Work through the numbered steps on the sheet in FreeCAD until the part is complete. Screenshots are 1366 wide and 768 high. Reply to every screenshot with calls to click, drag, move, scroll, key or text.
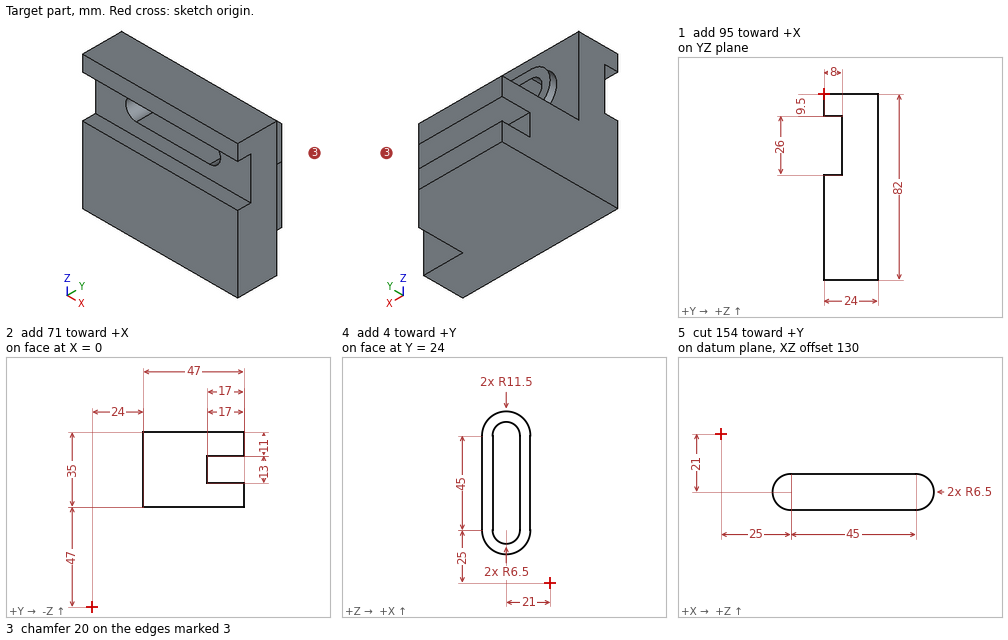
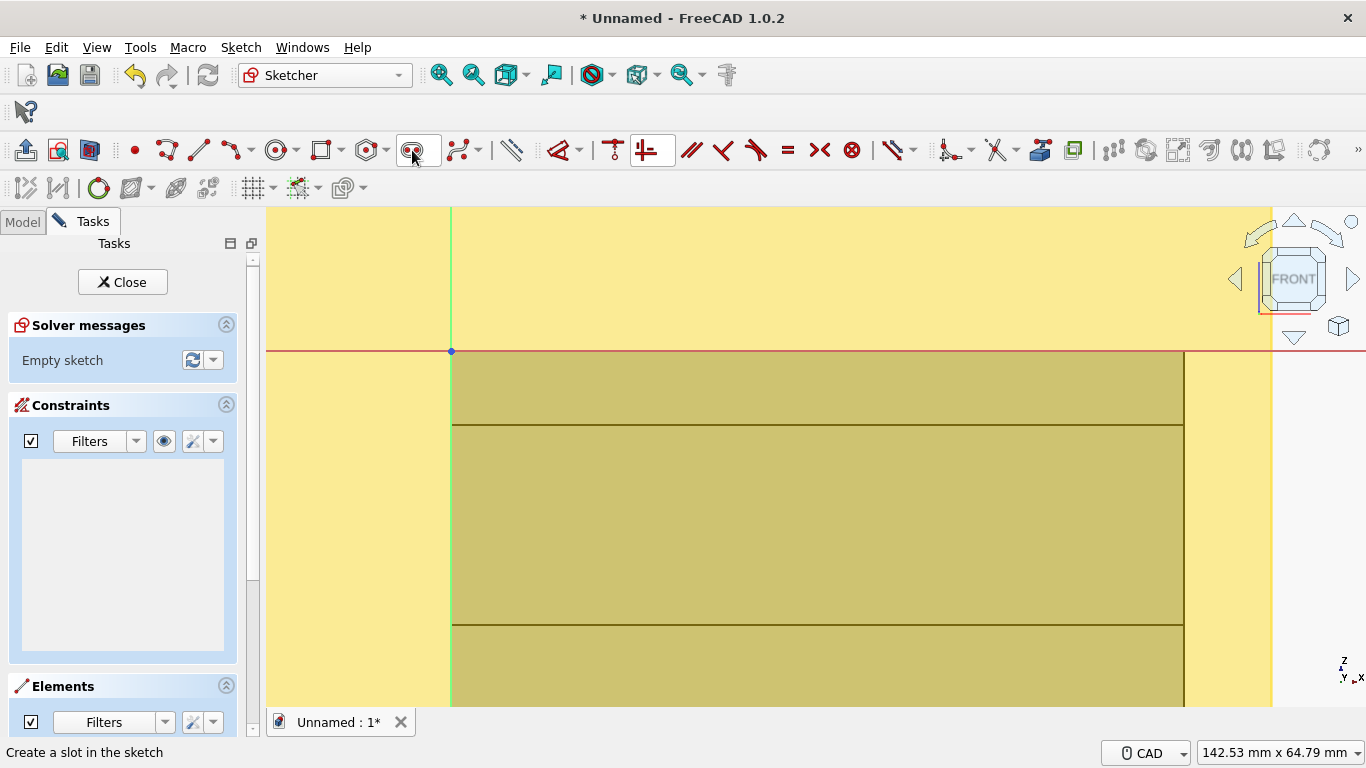
click(644, 513)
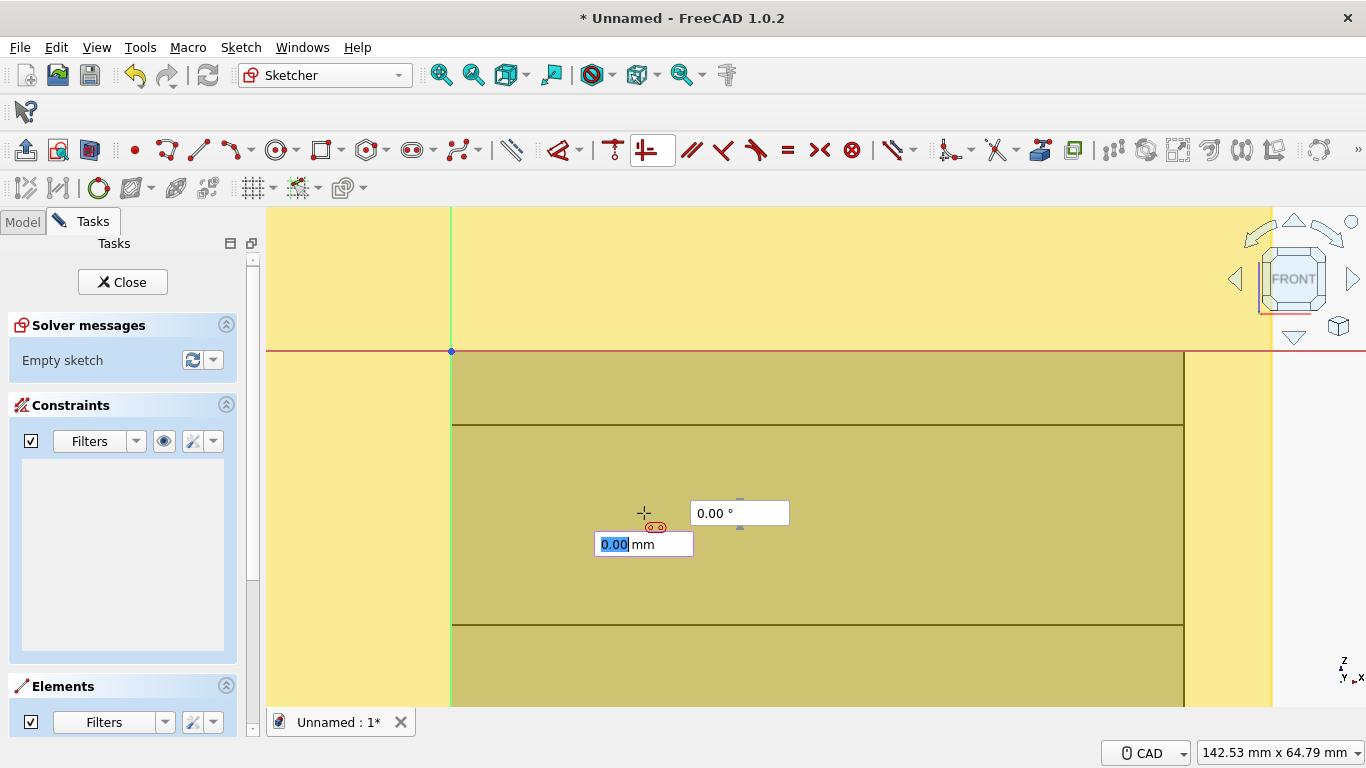
click(991, 513)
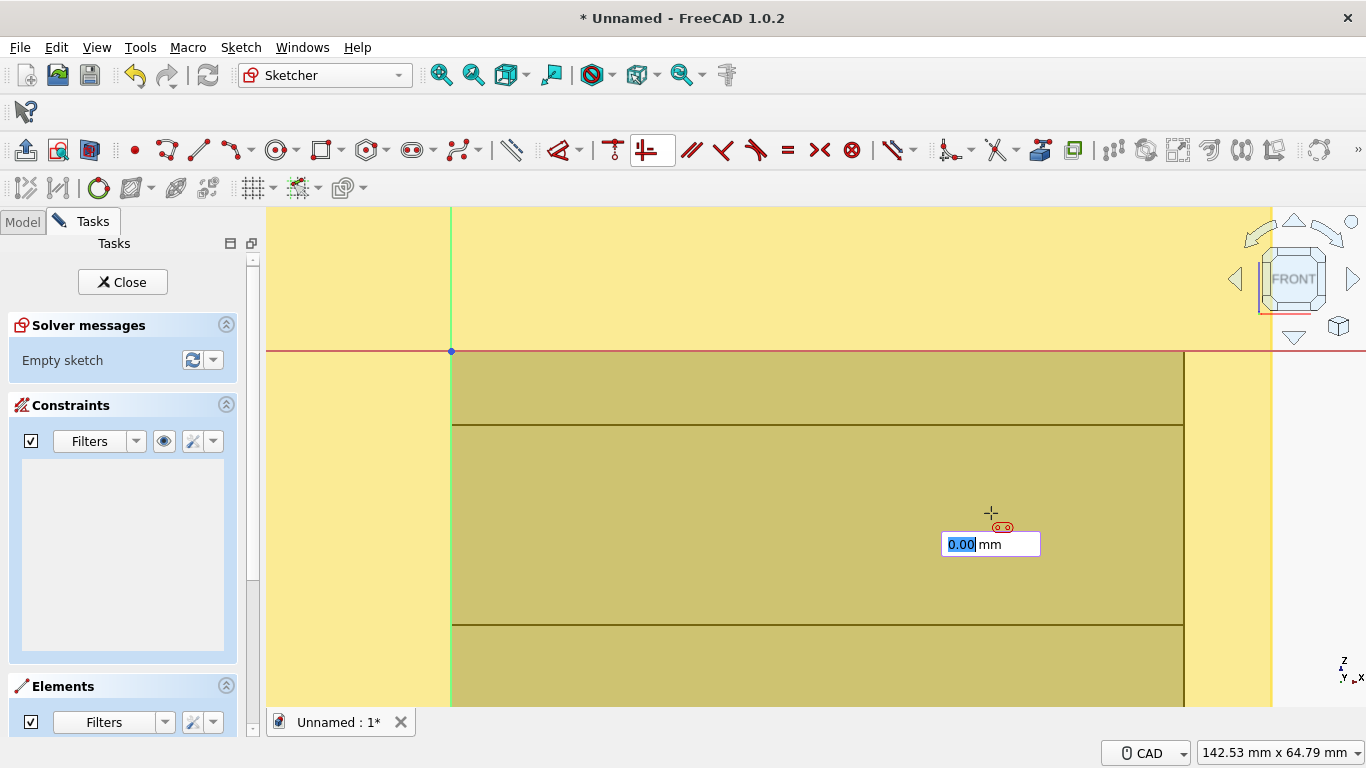
click(818, 563)
key(Escape)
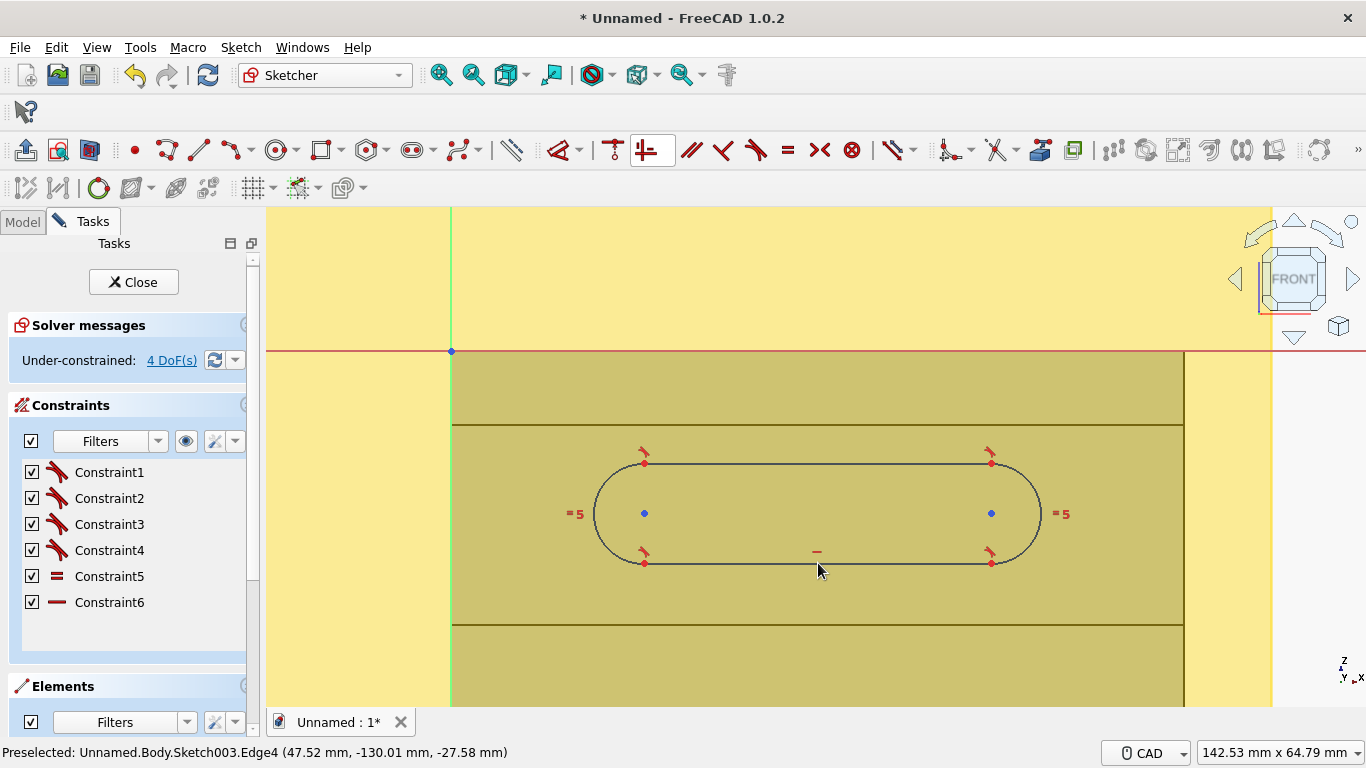
click(558, 150)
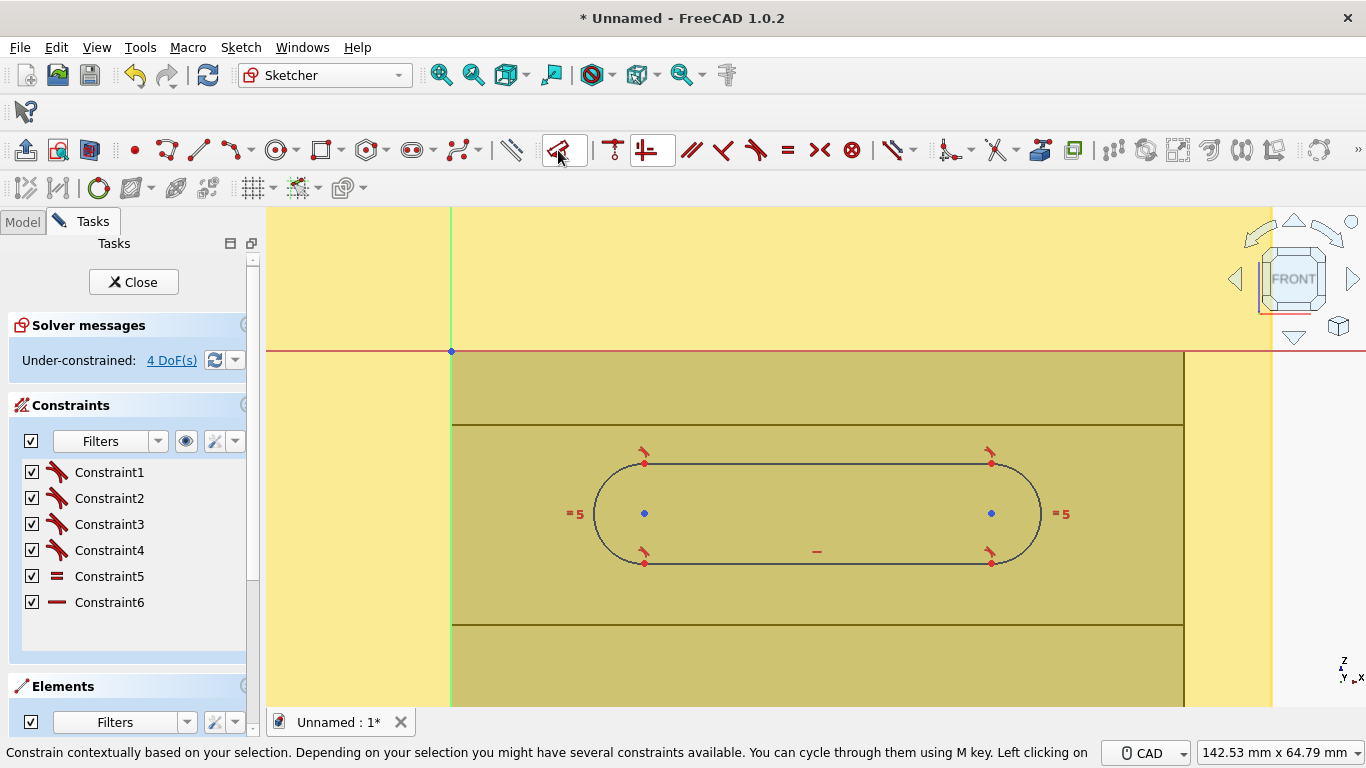
click(604, 485)
click(578, 466)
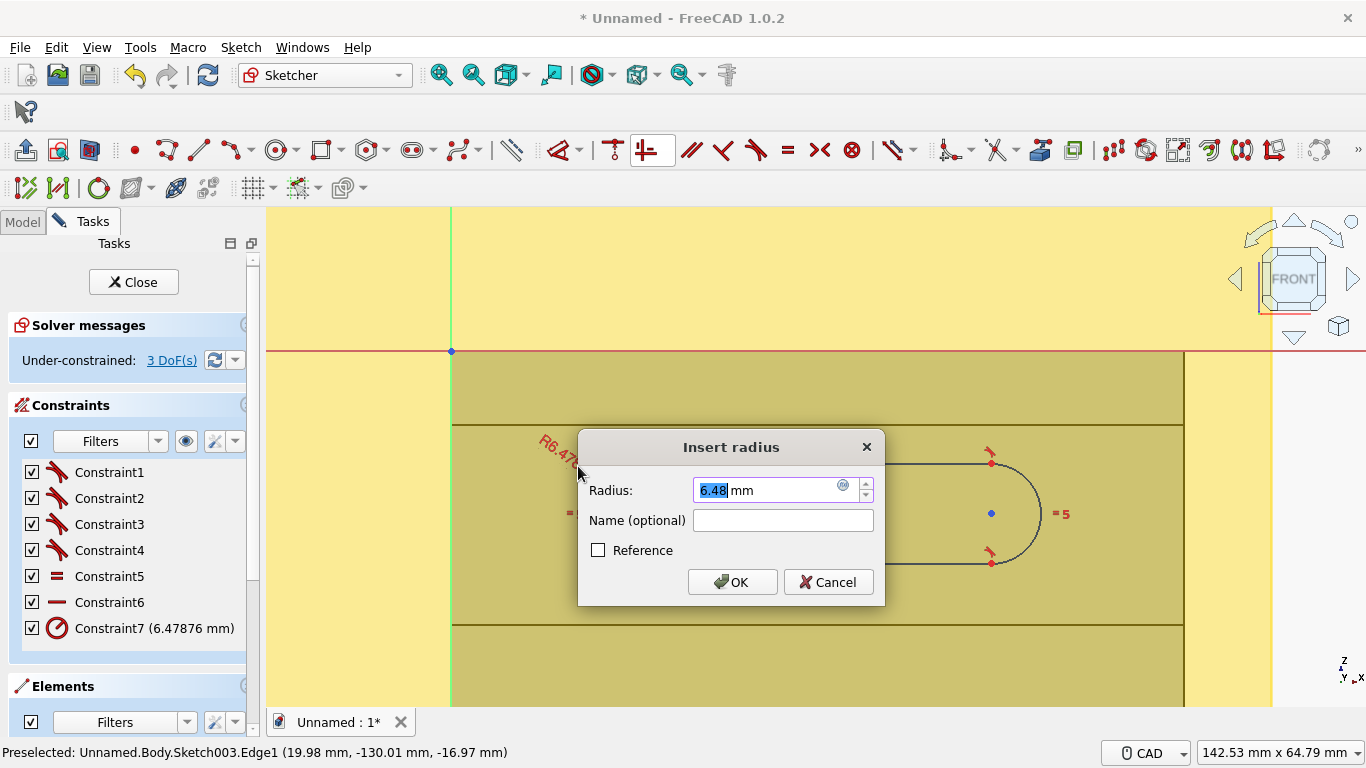
text(6.5)
key(Return)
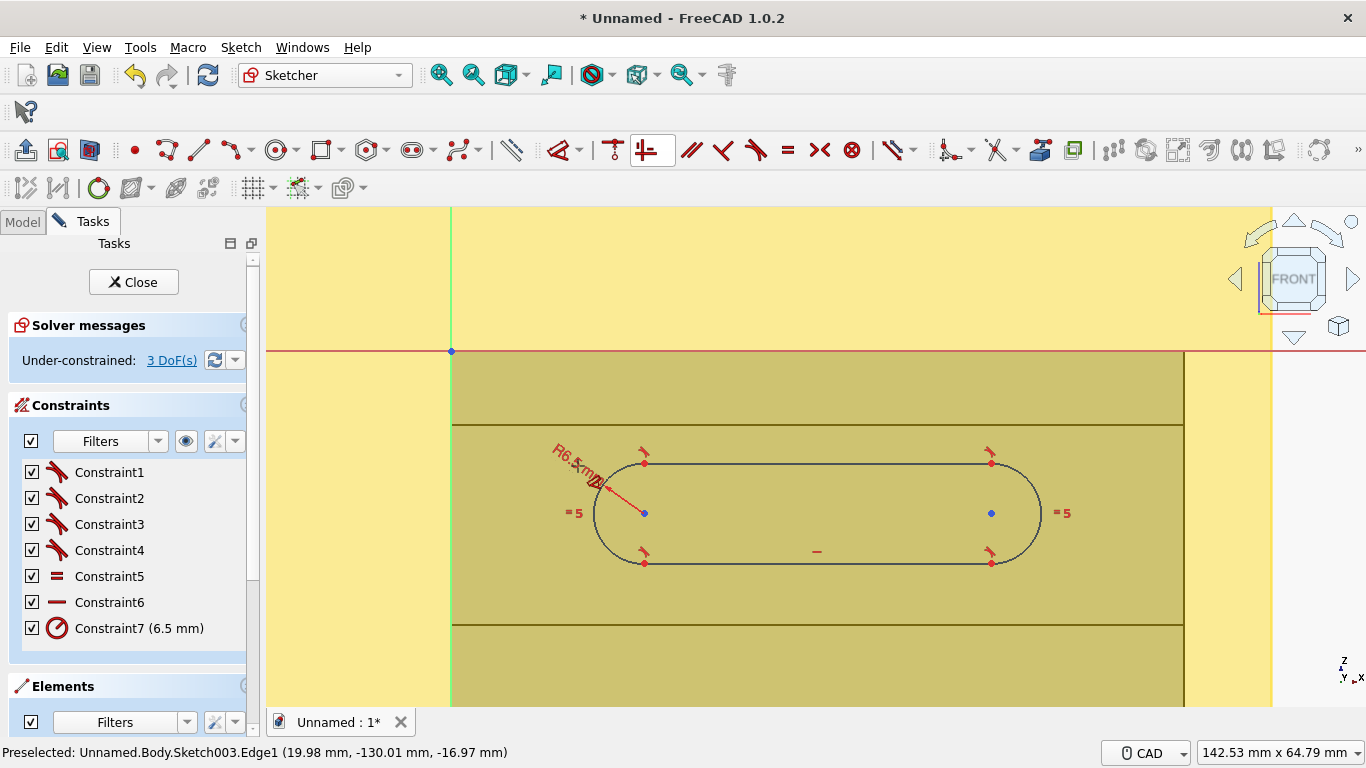
click(748, 464)
click(818, 498)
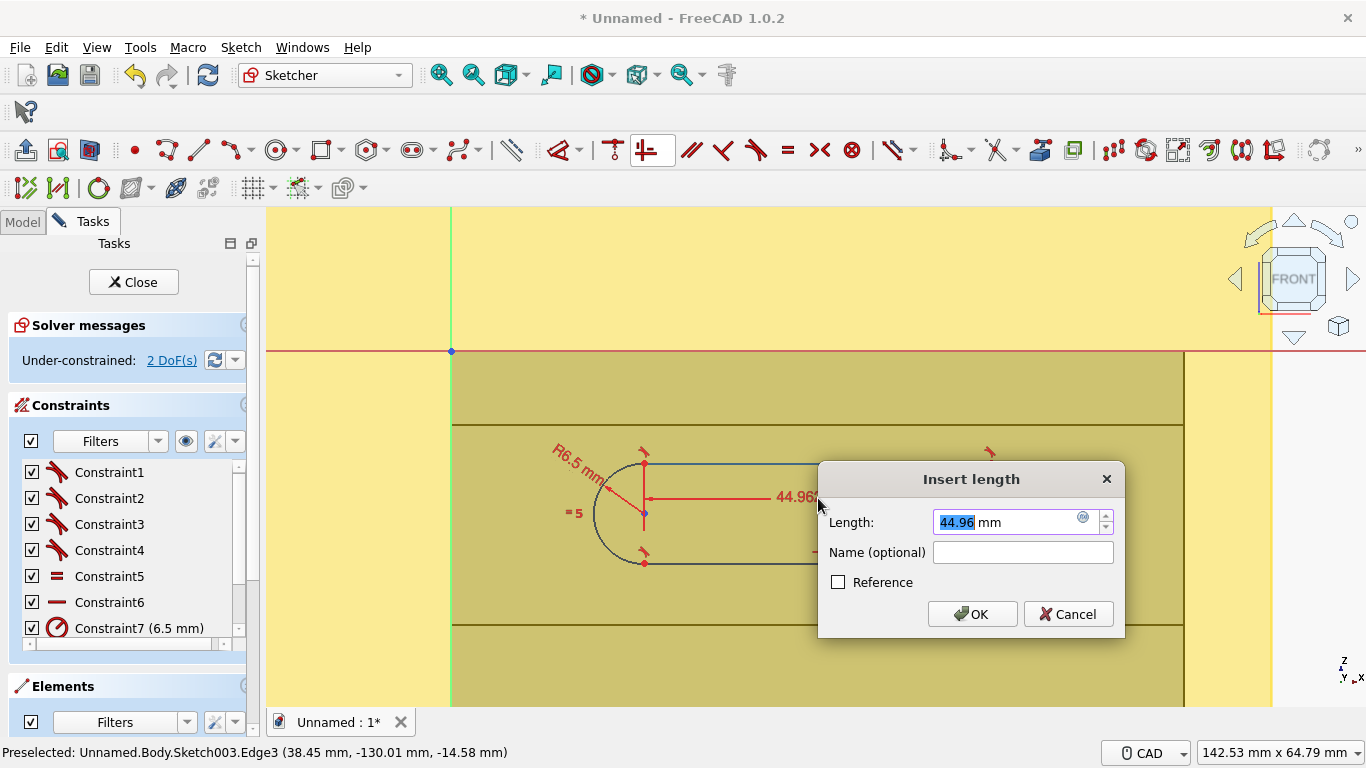
text(45)
key(Return)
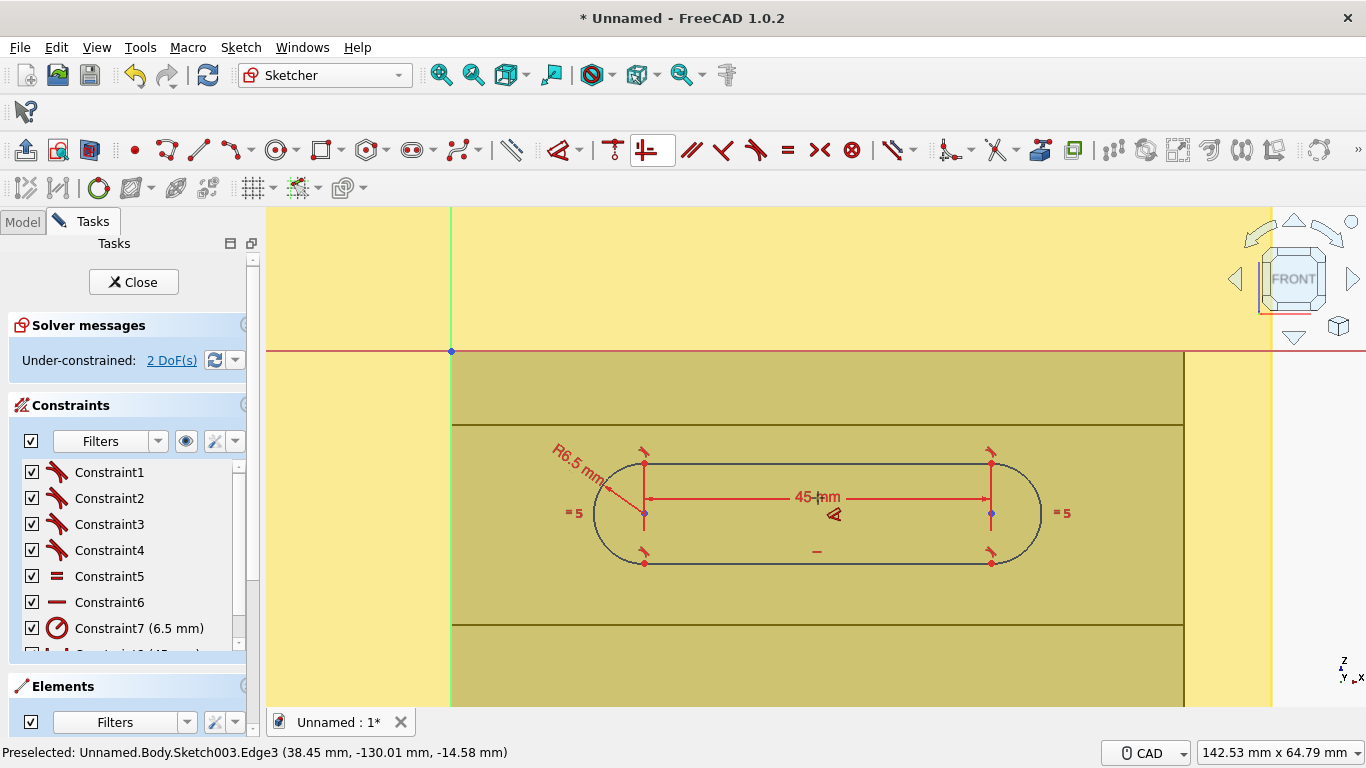
click(644, 464)
click(548, 317)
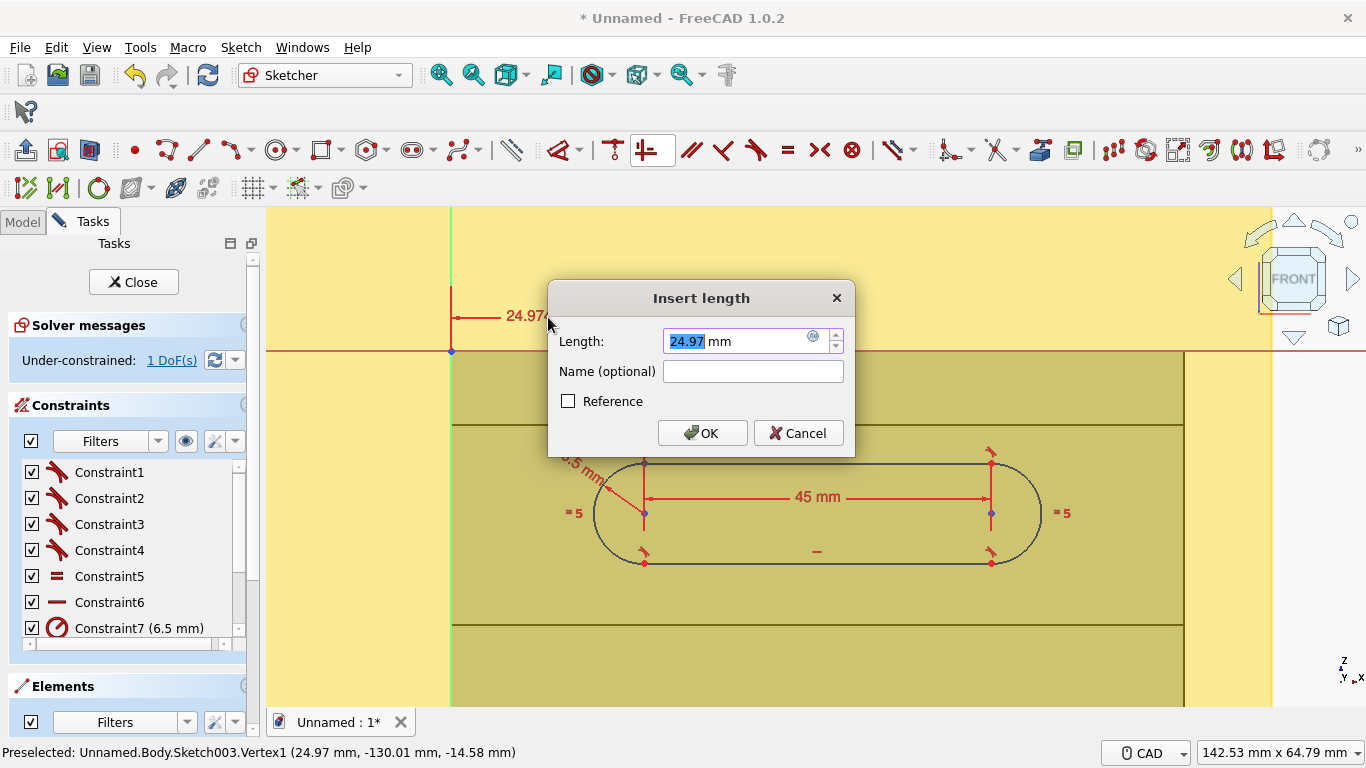
text(25)
key(Return)